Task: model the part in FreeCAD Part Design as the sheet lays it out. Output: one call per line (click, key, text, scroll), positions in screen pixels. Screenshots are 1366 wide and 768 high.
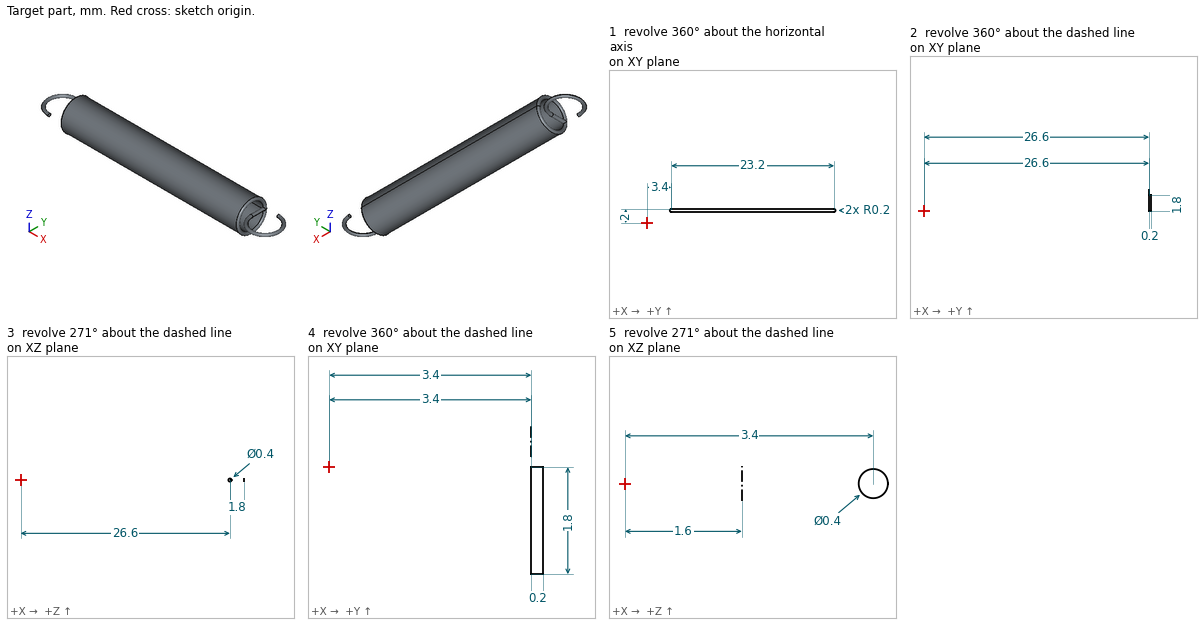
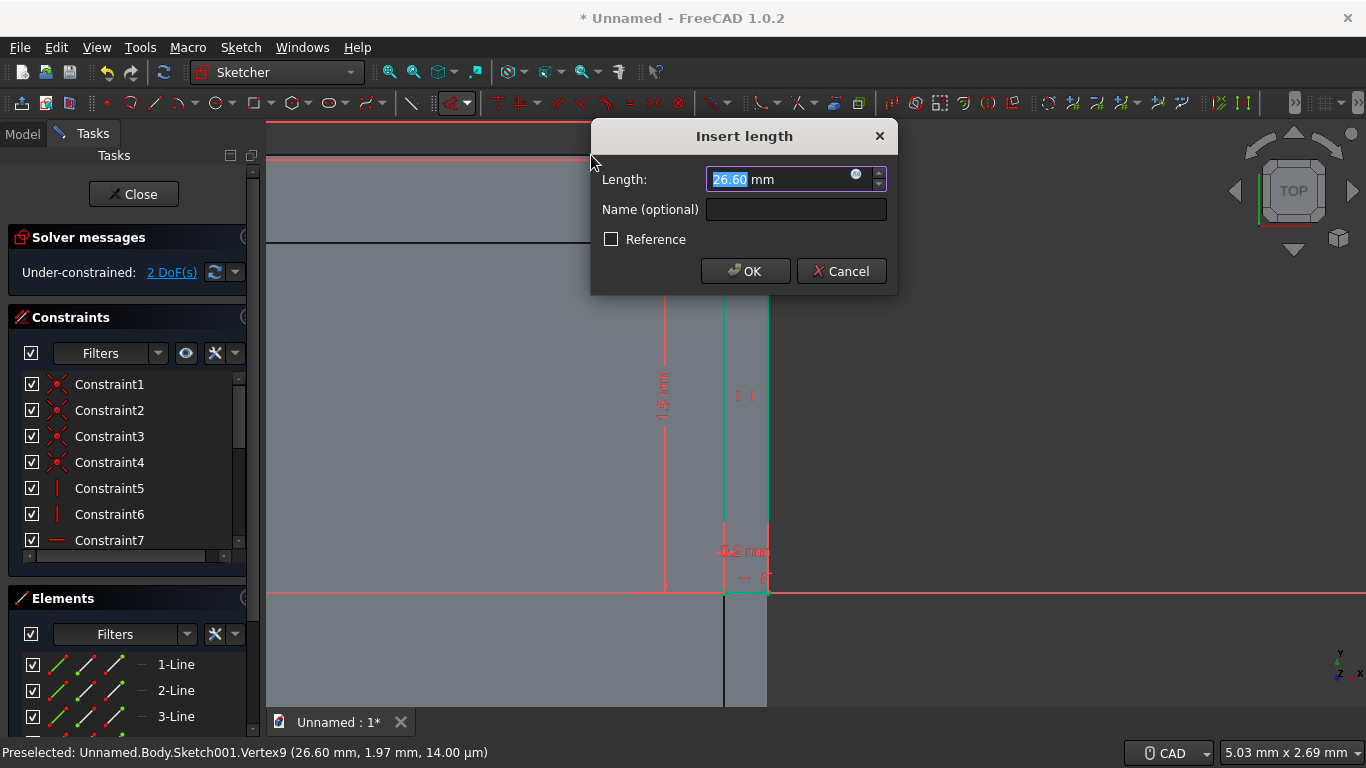
text(26.6)
key(Return)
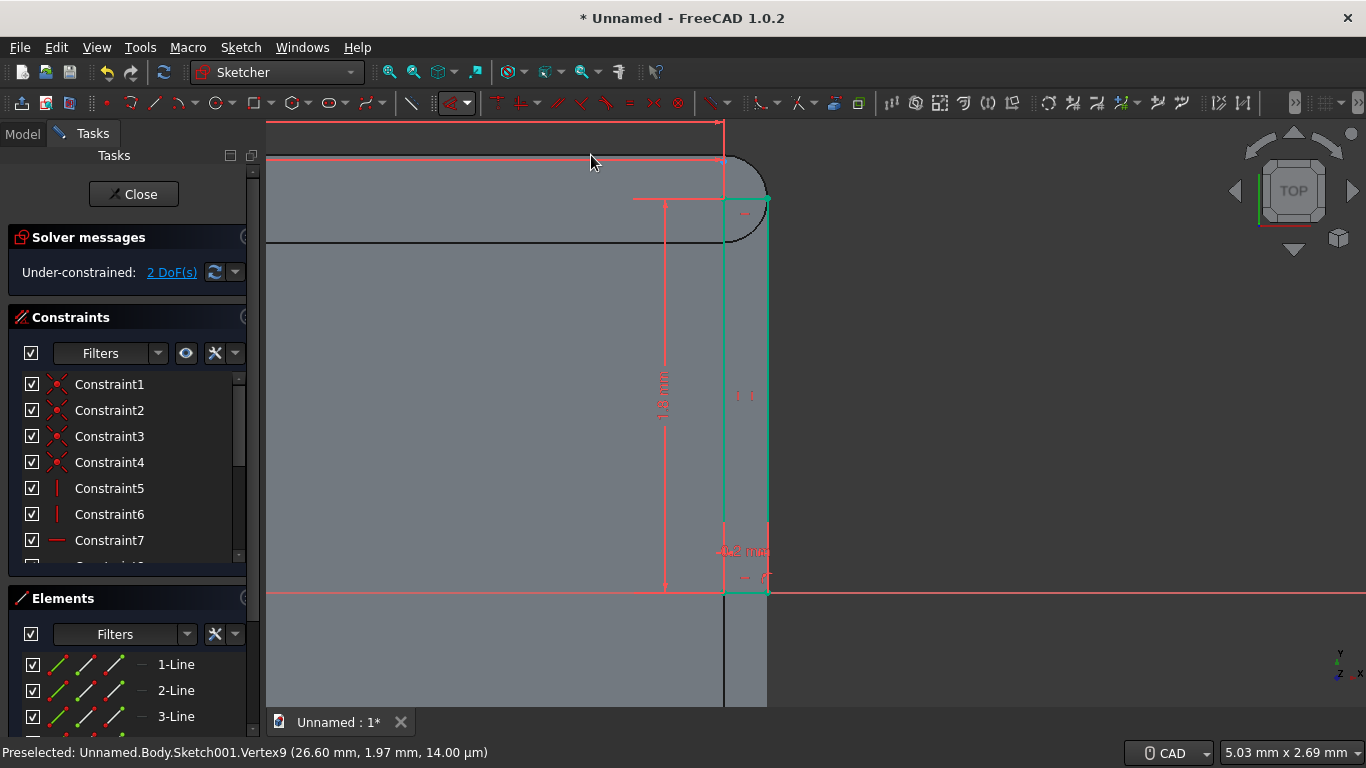
click(134, 194)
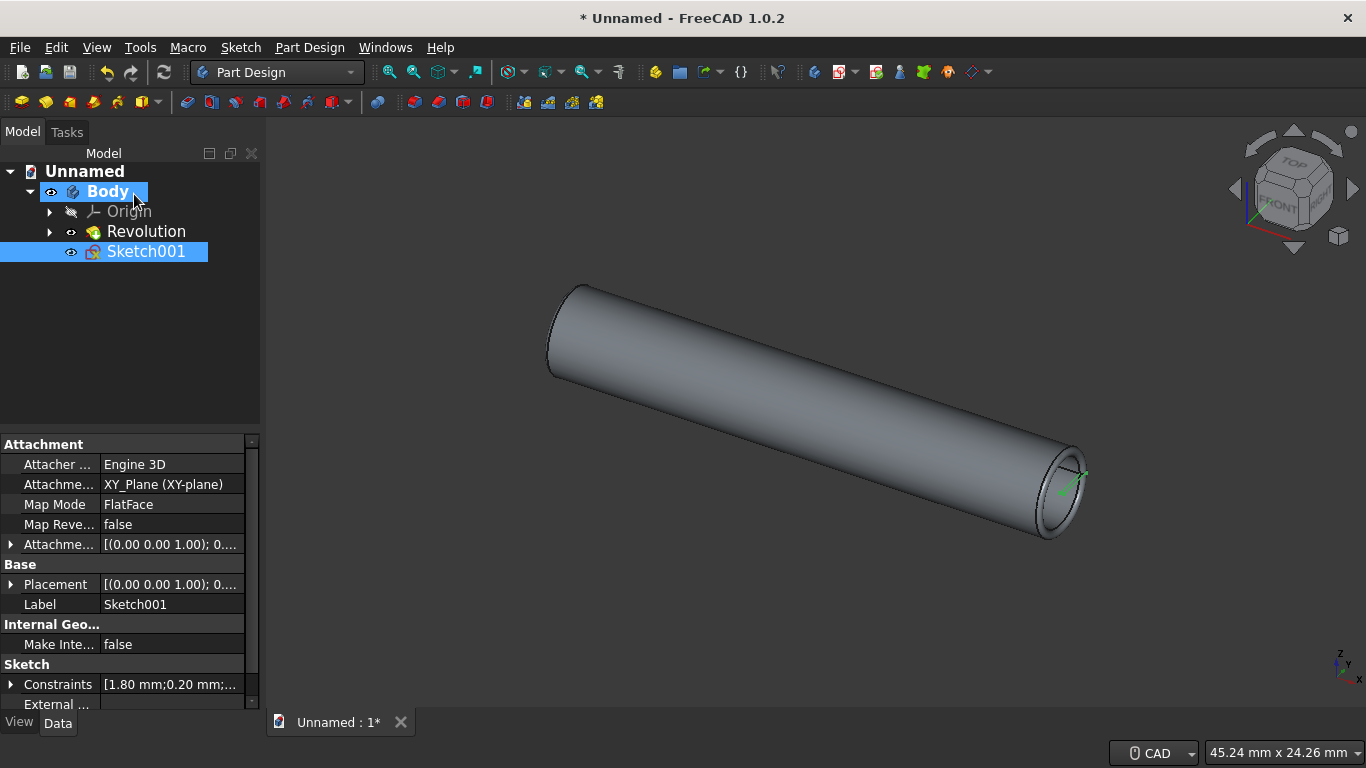
click(46, 102)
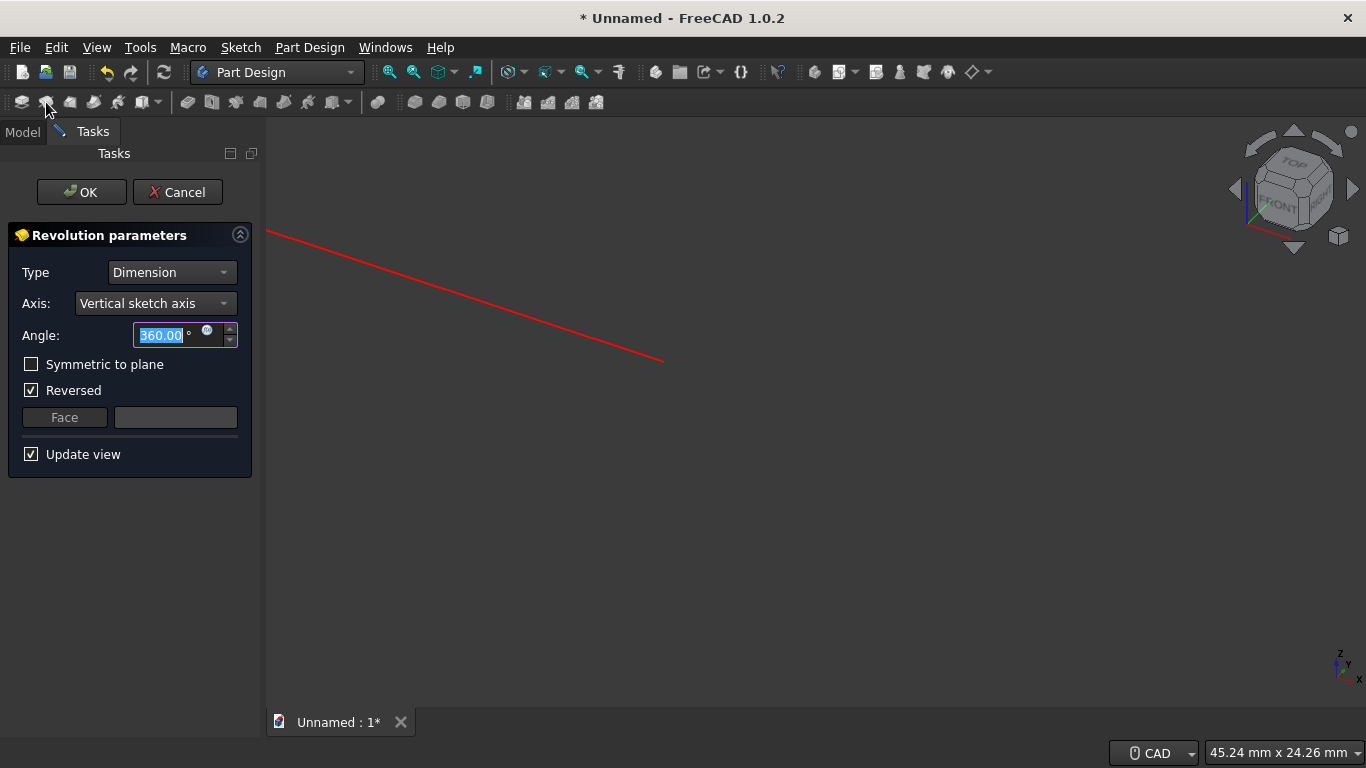
click(156, 304)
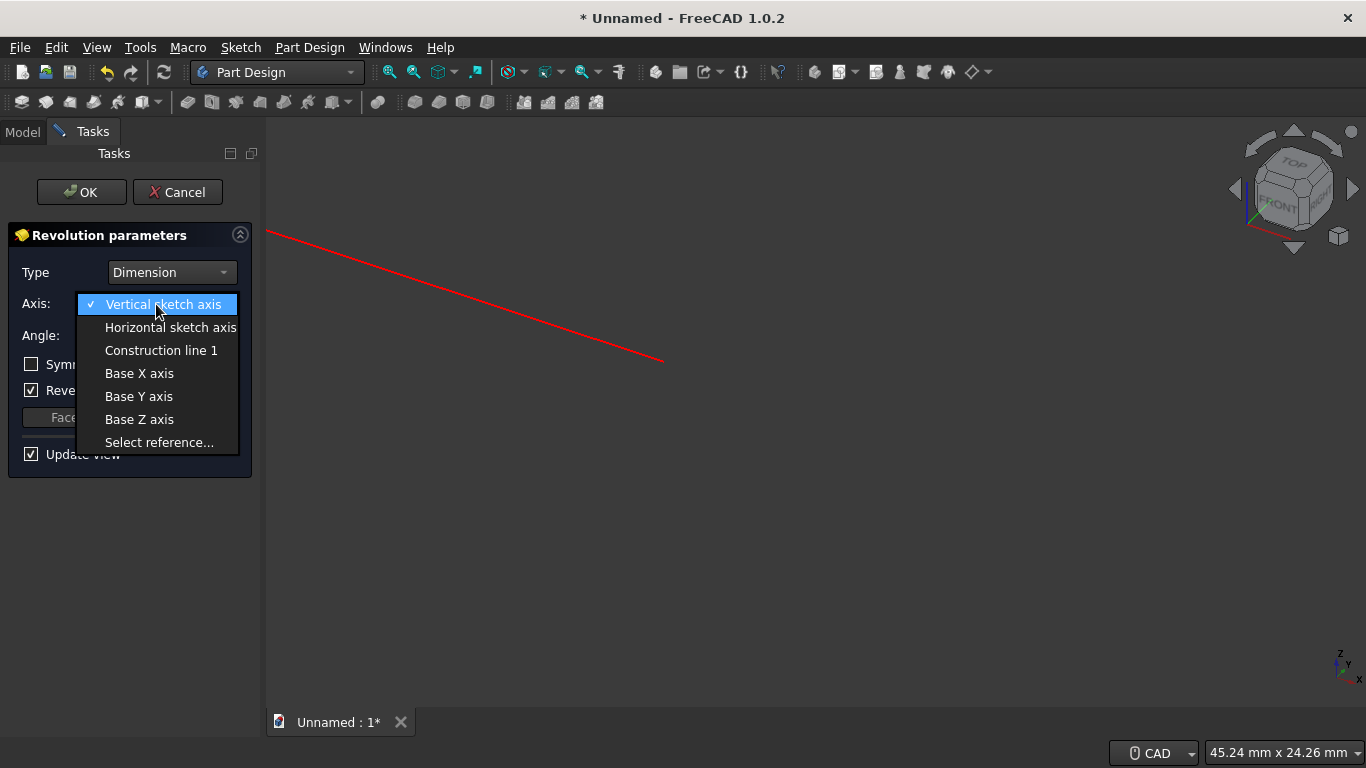
click(156, 350)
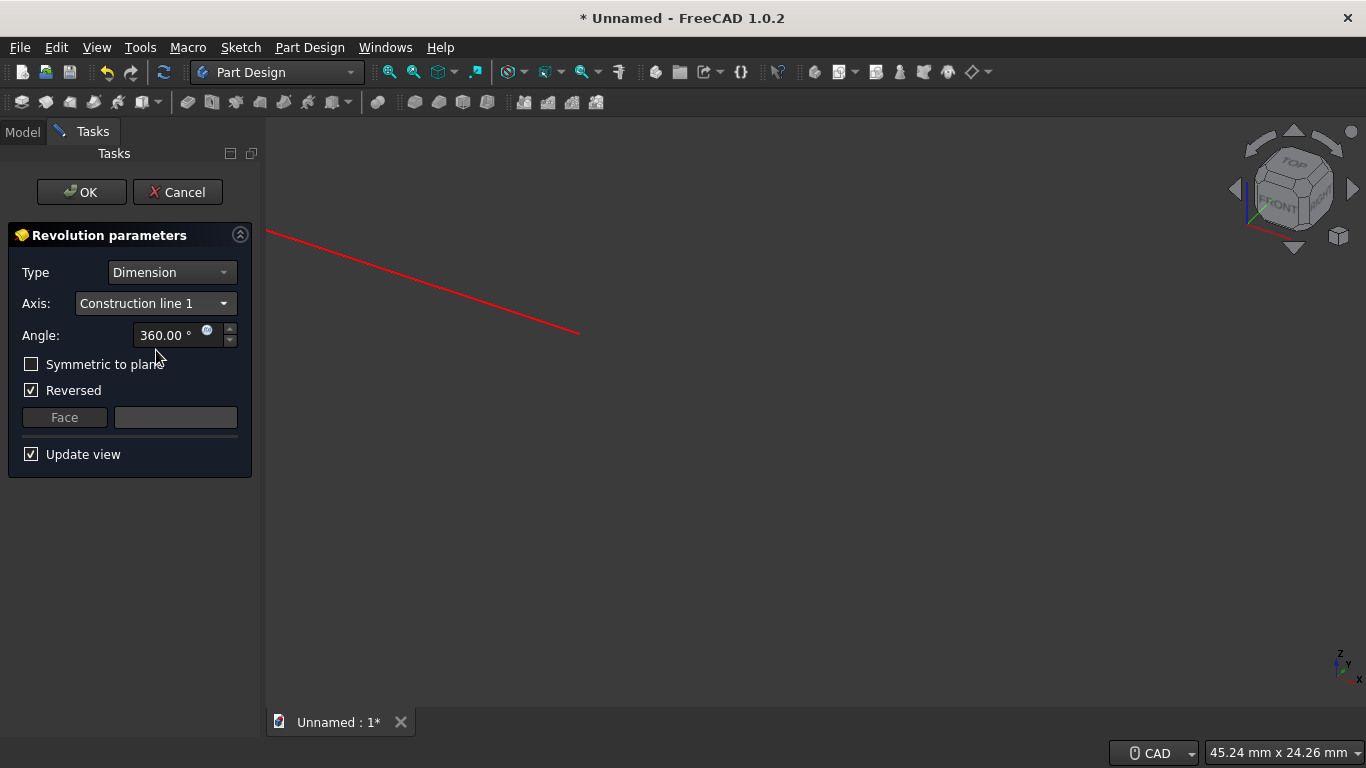
click(82, 192)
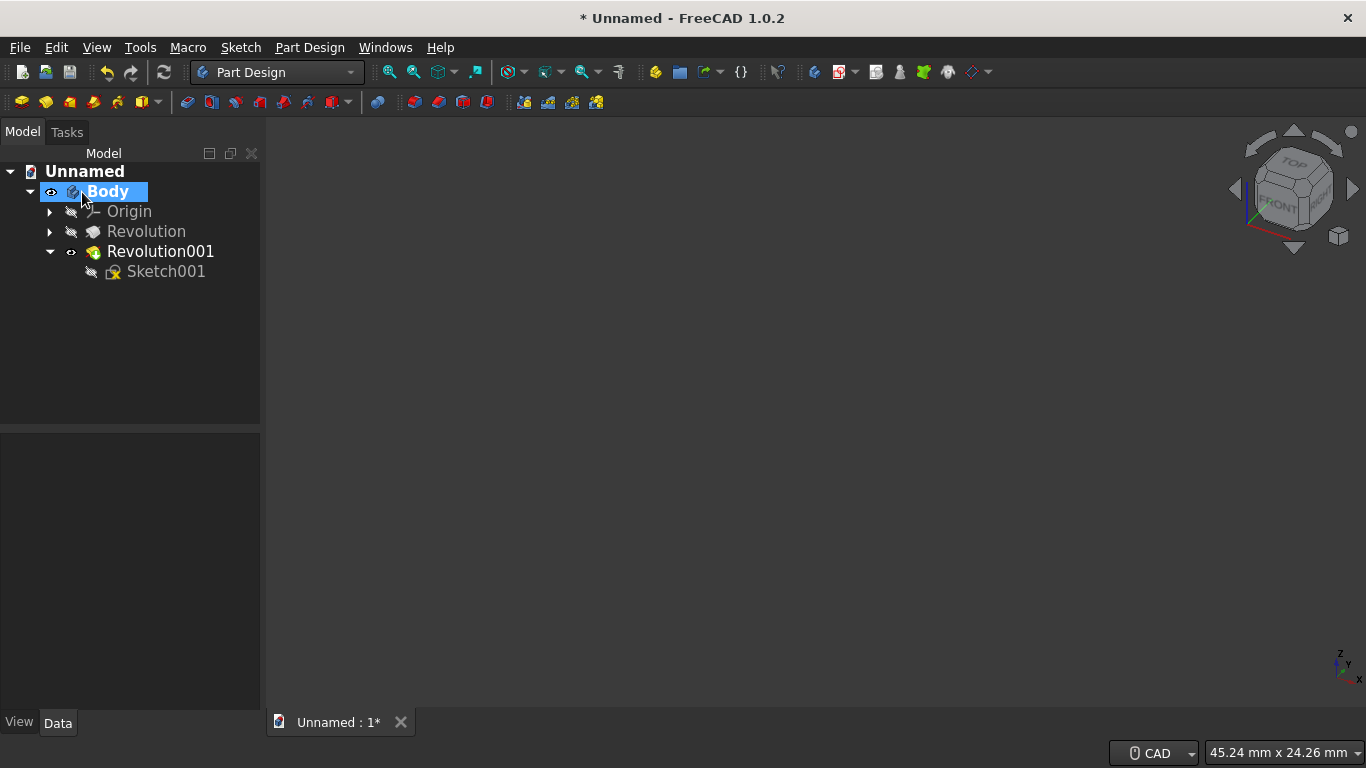
click(390, 72)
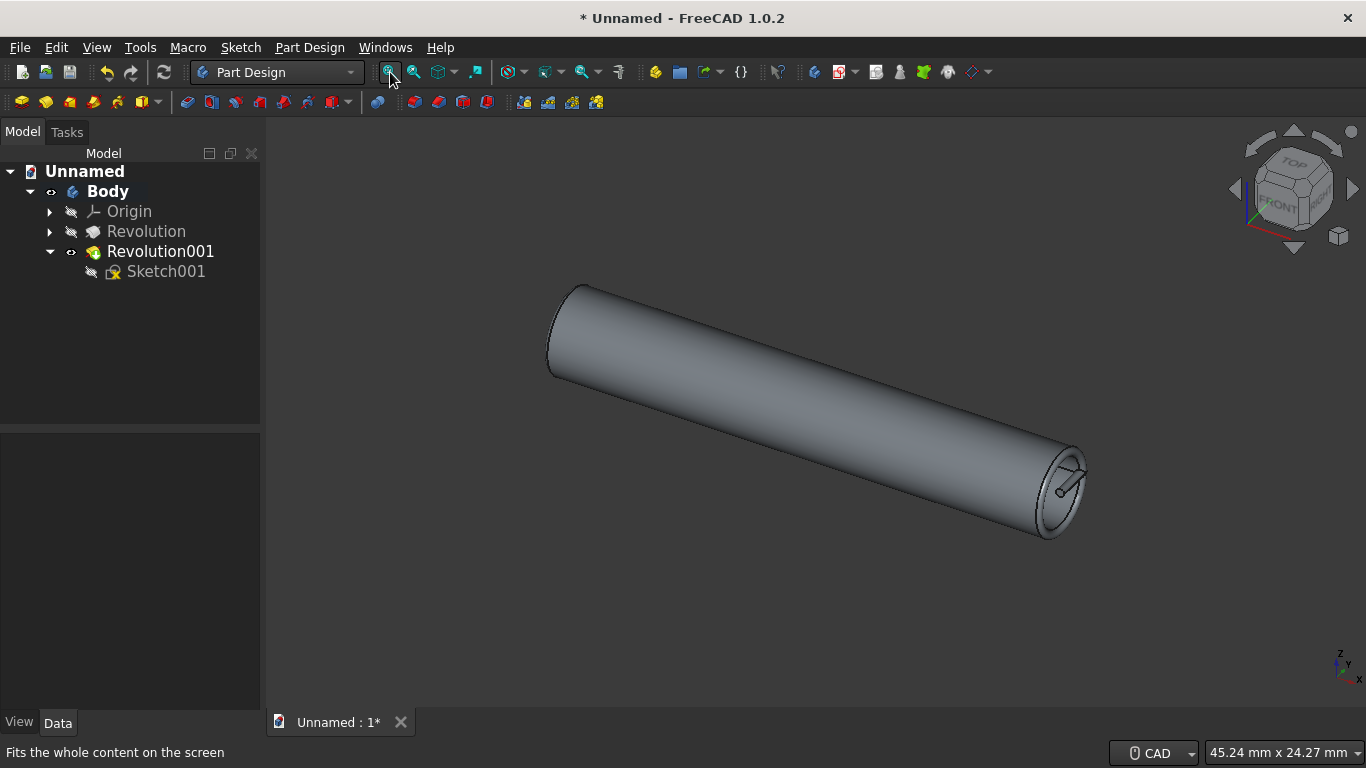
click(840, 72)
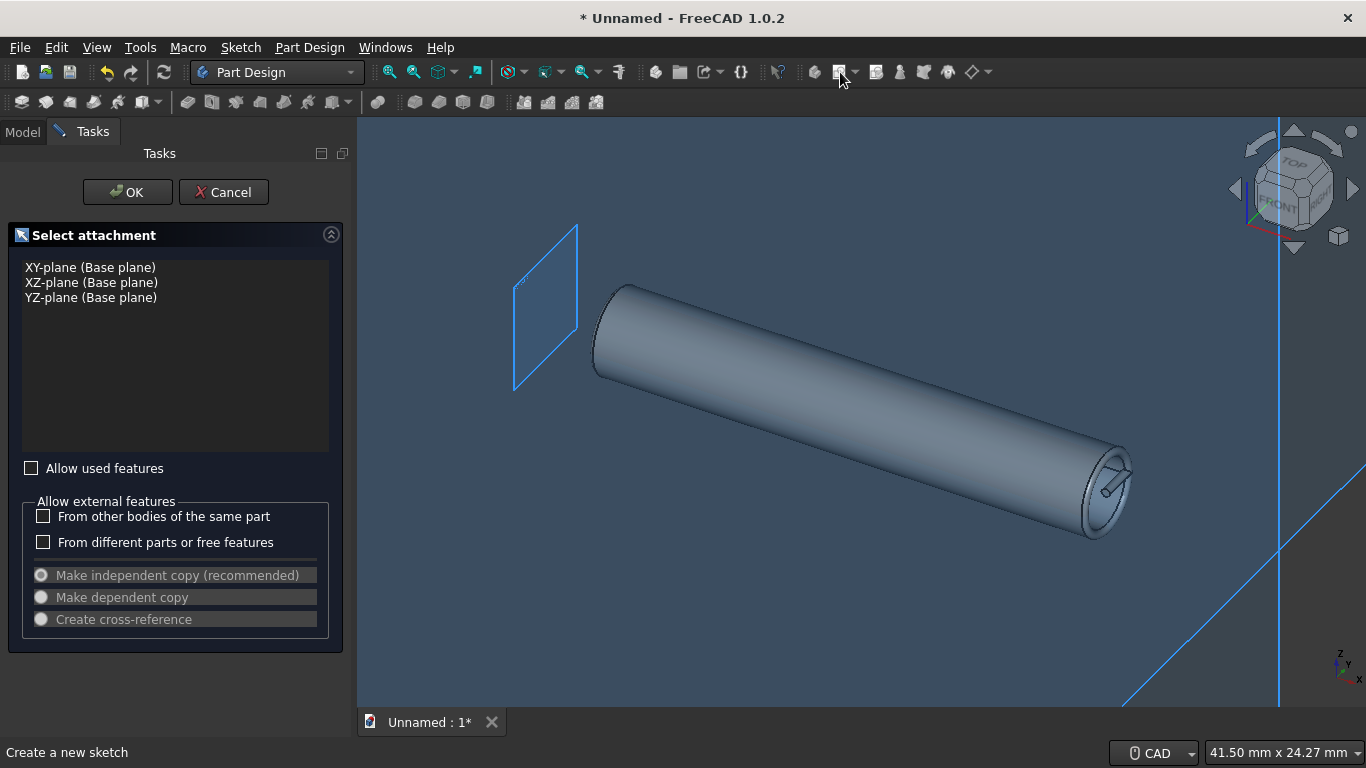
click(82, 282)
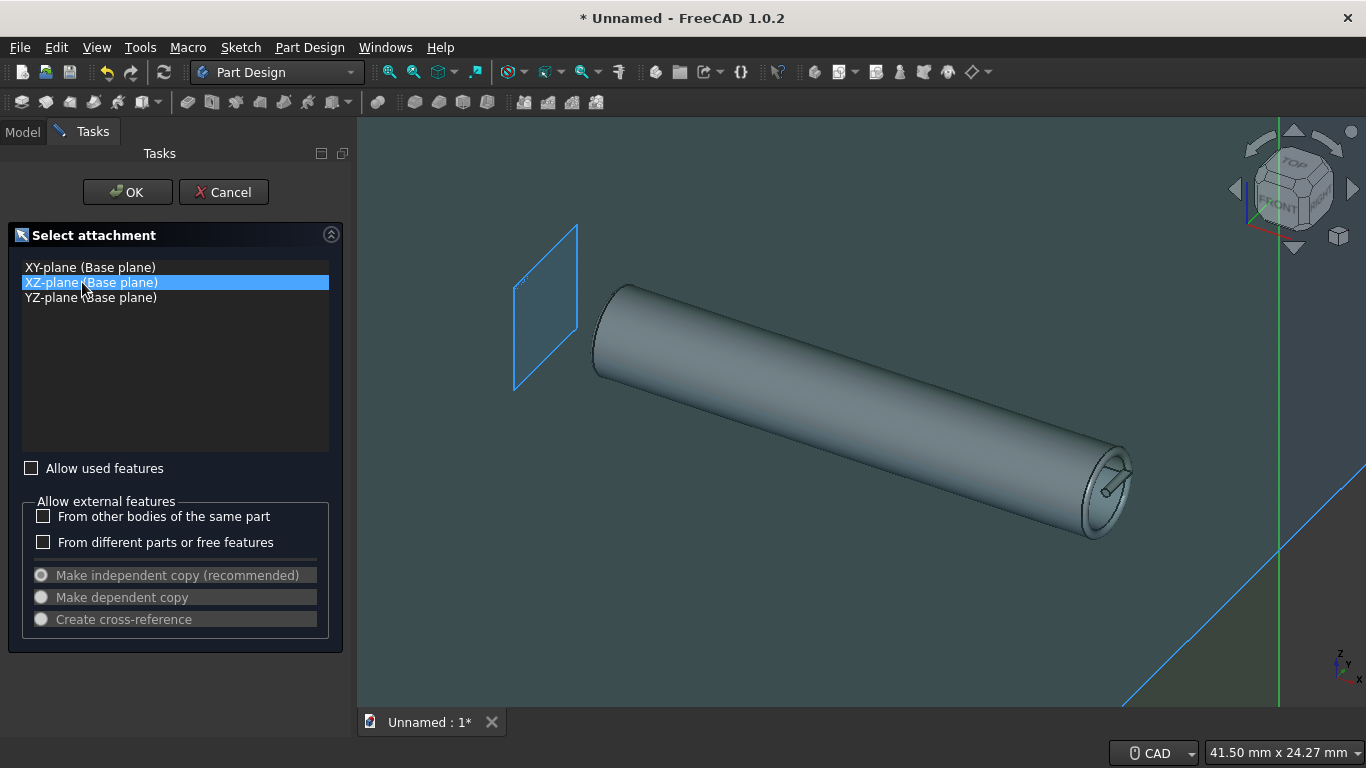
click(128, 192)